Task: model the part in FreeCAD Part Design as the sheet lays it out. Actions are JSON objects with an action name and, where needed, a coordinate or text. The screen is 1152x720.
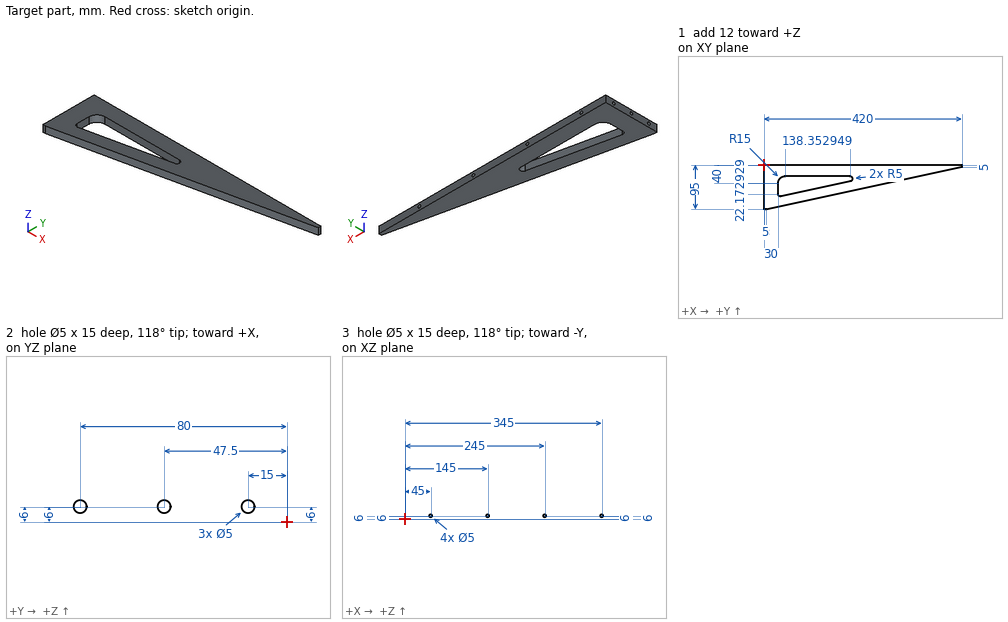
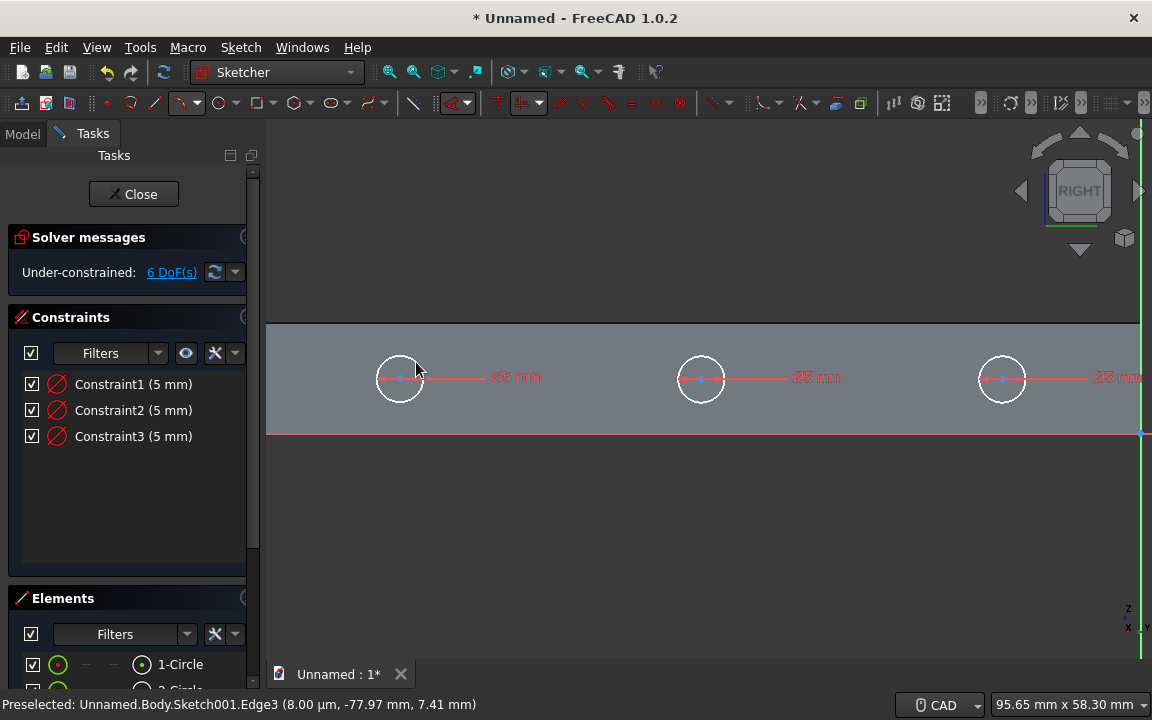
{"action": "scroll", "coordinate": [400, 378], "scroll_direction": "down", "scroll_amount": 2}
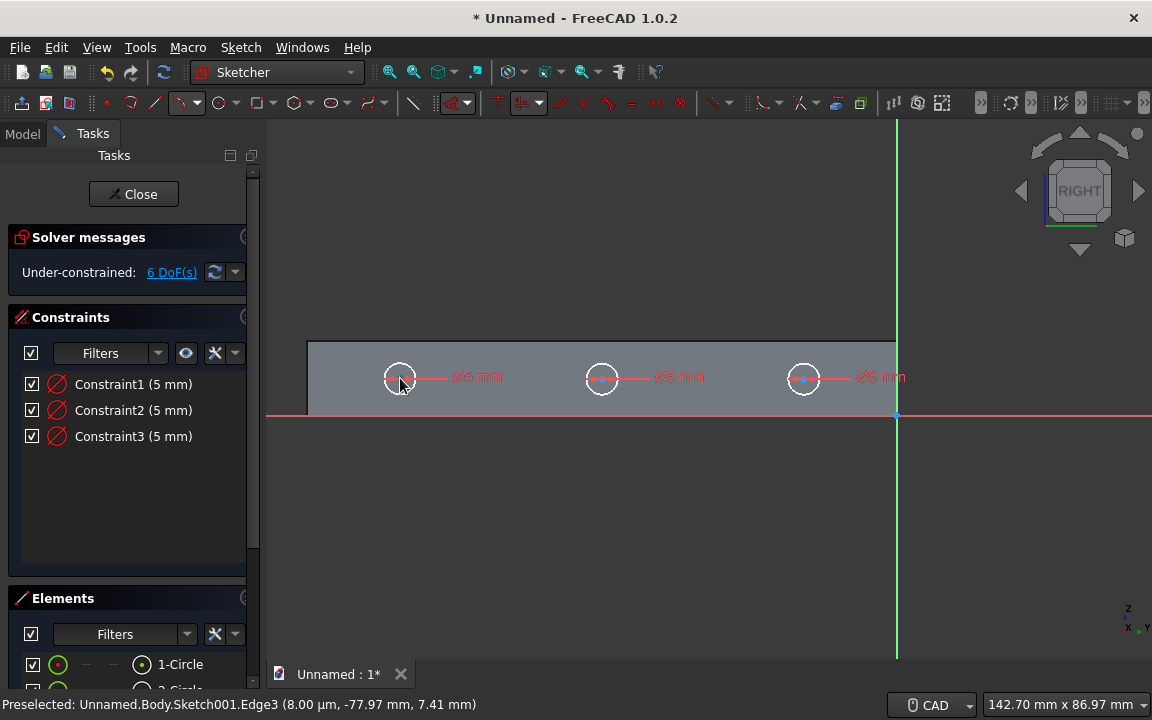
{"action": "left_click", "coordinate": [804, 379]}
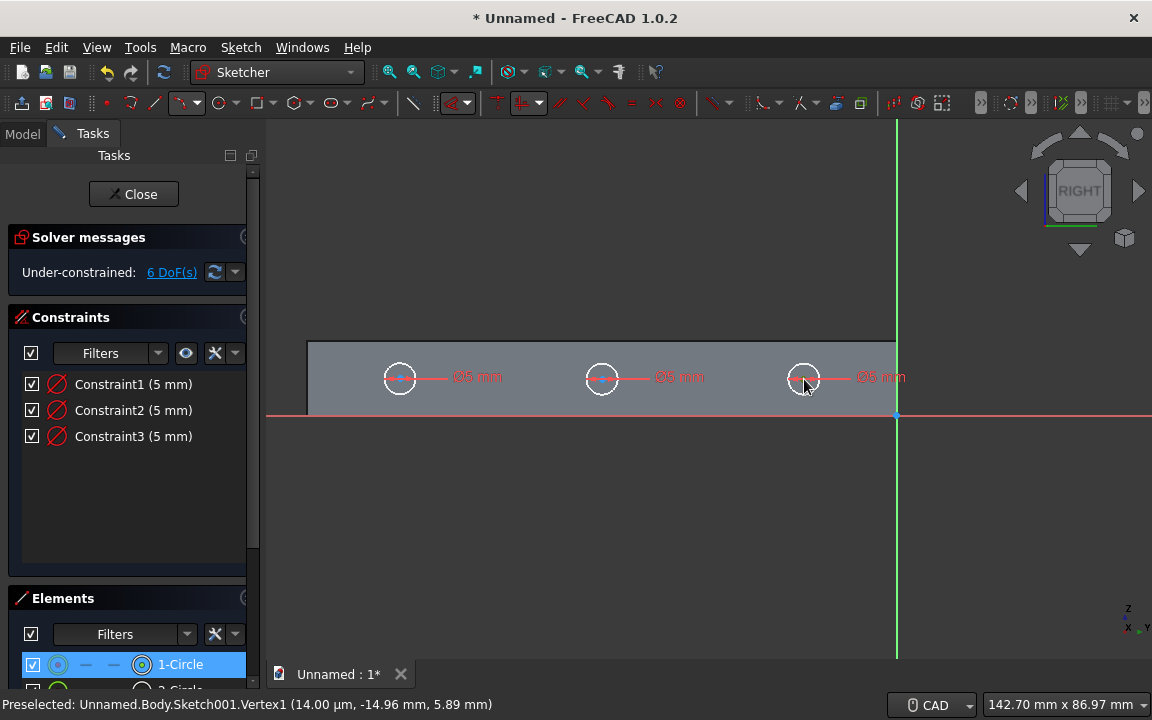
{"action": "left_click", "coordinate": [470, 104]}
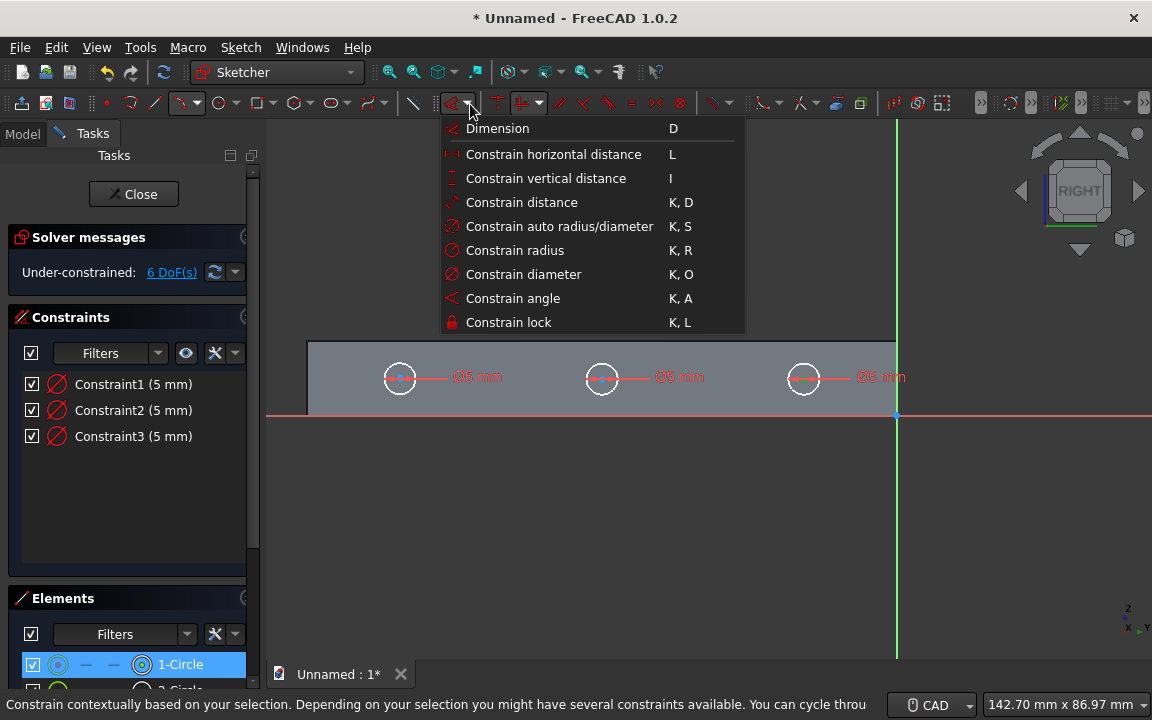
{"action": "left_click", "coordinate": [593, 178]}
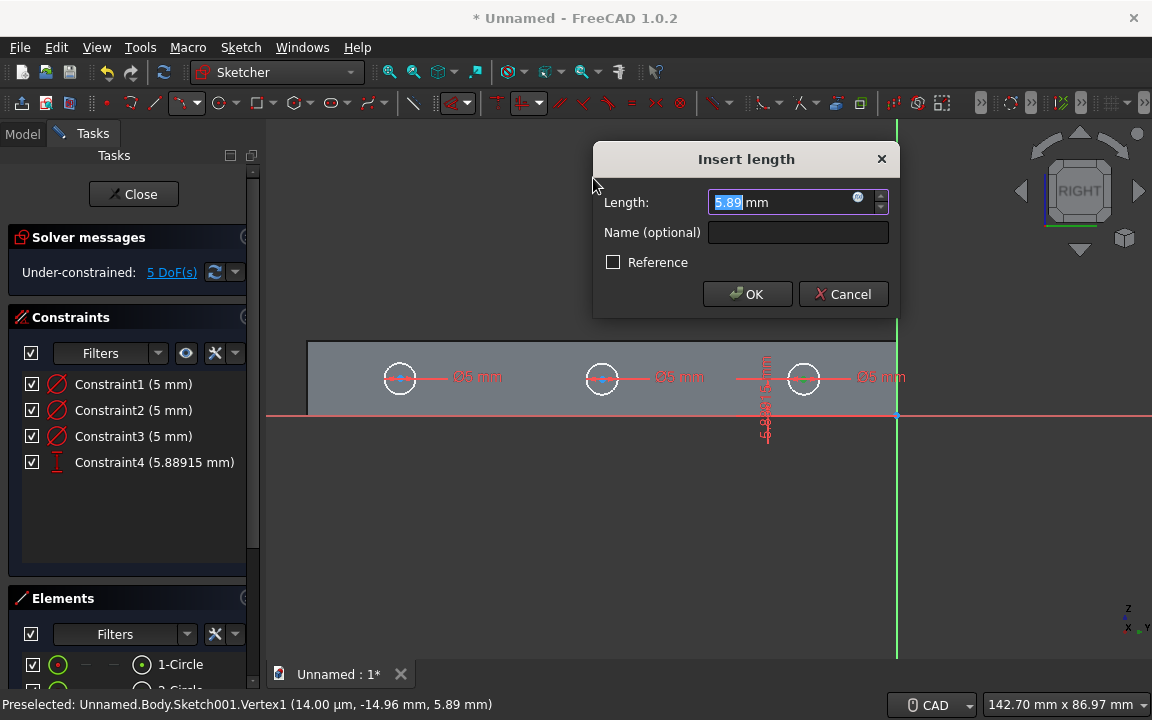
{"action": "type", "text": "6"}
{"action": "key", "text": "Return"}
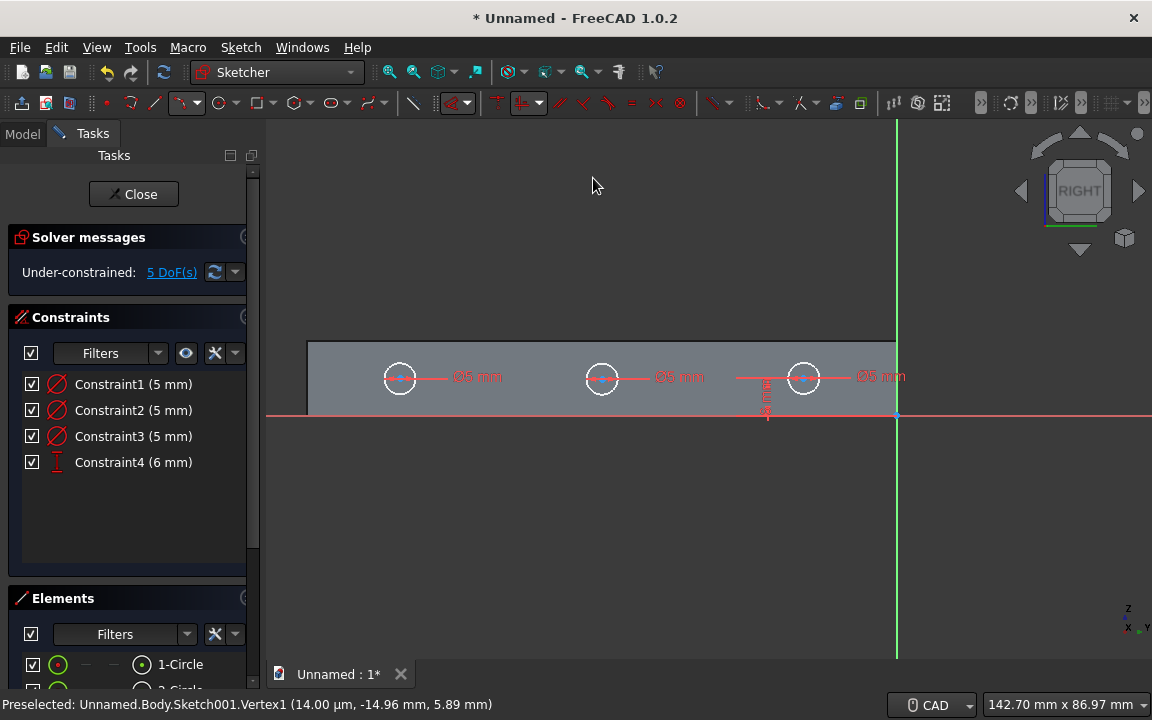
{"action": "left_click", "coordinate": [602, 379]}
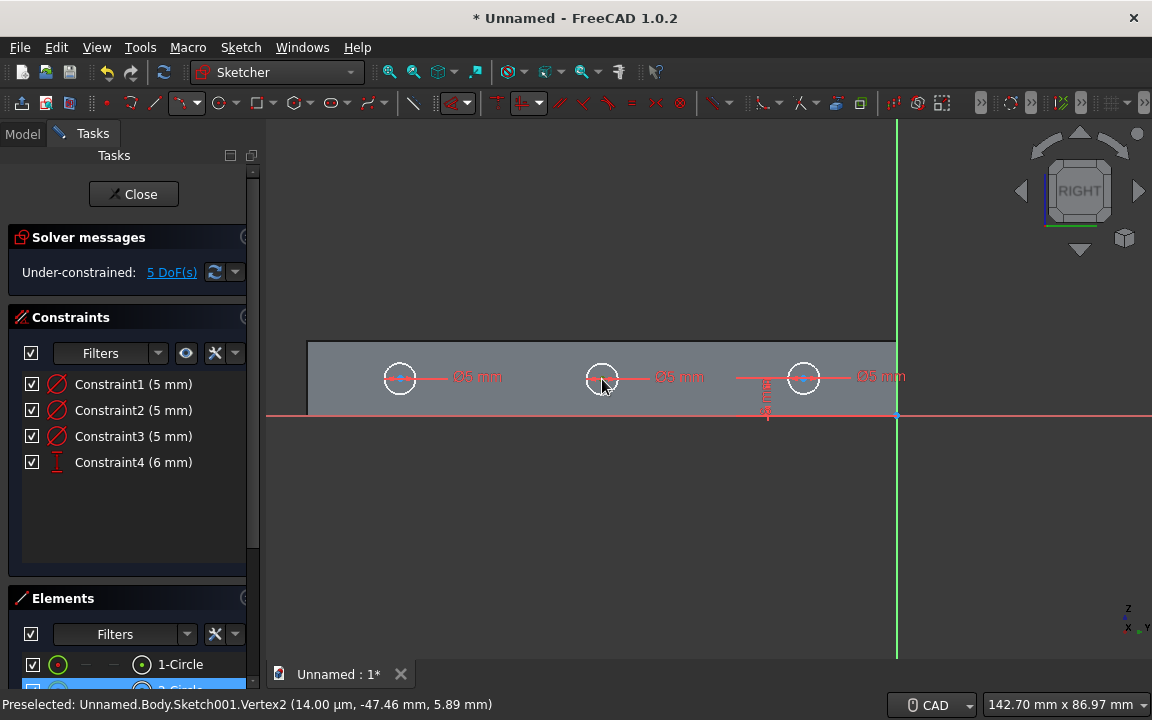
{"action": "left_click", "coordinate": [470, 104]}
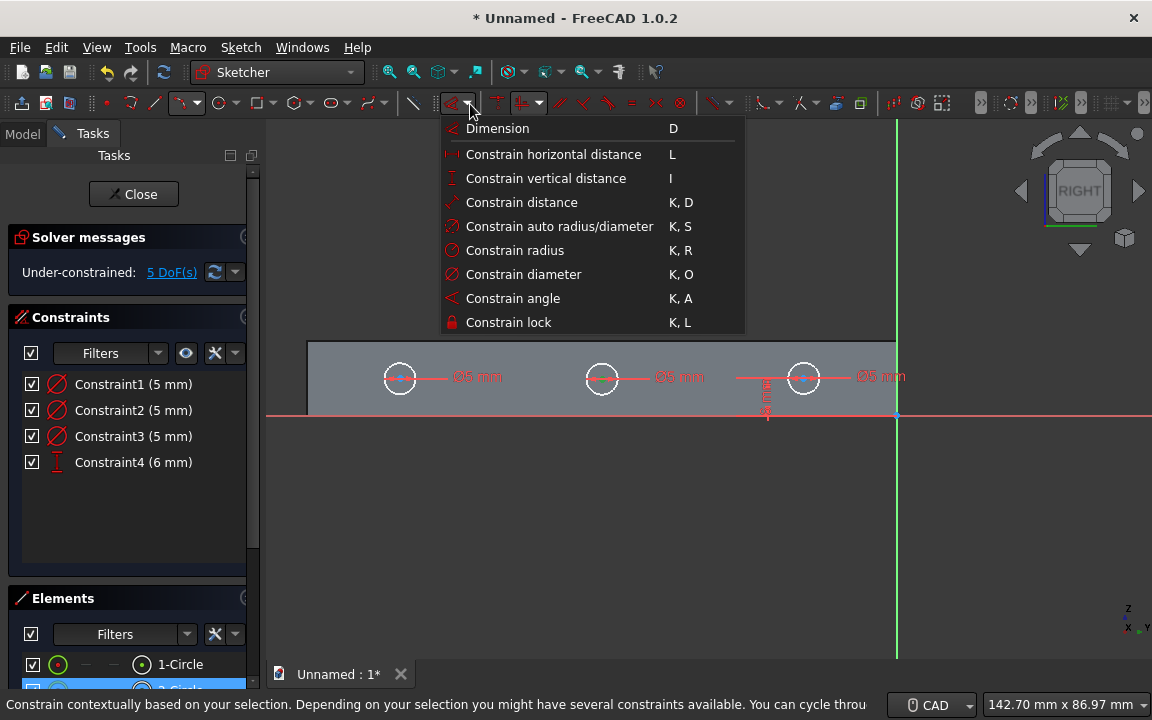
{"action": "left_click", "coordinate": [593, 178]}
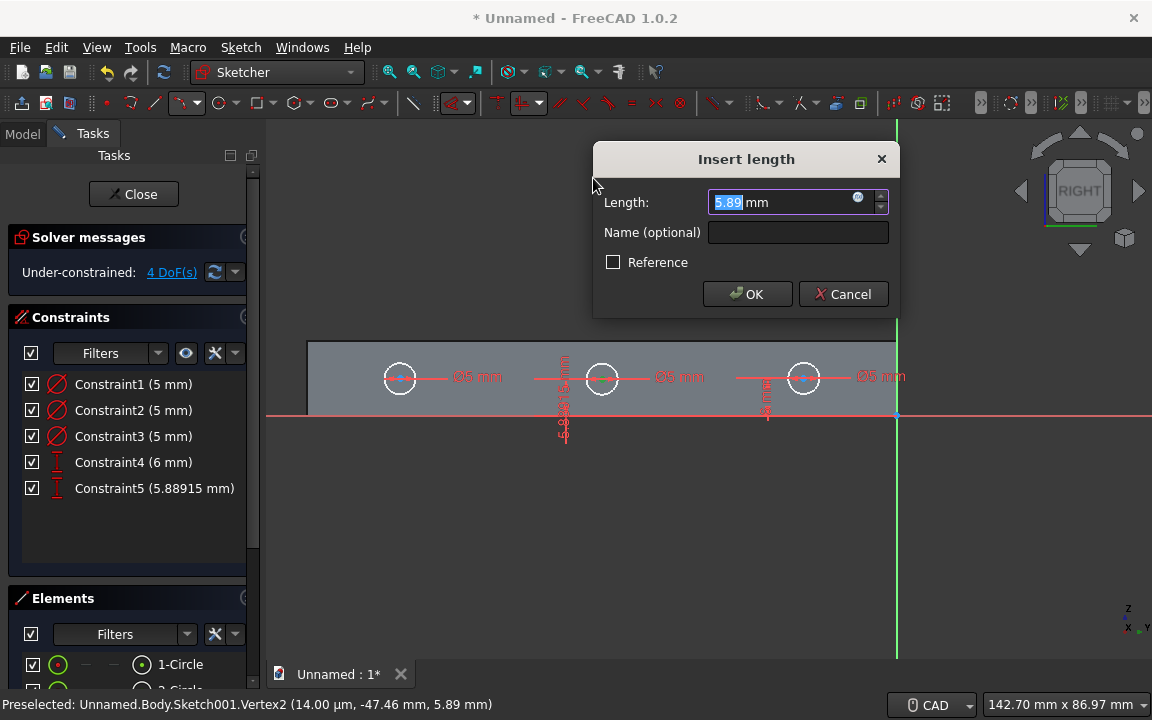
{"action": "type", "text": "6"}
{"action": "key", "text": "Return"}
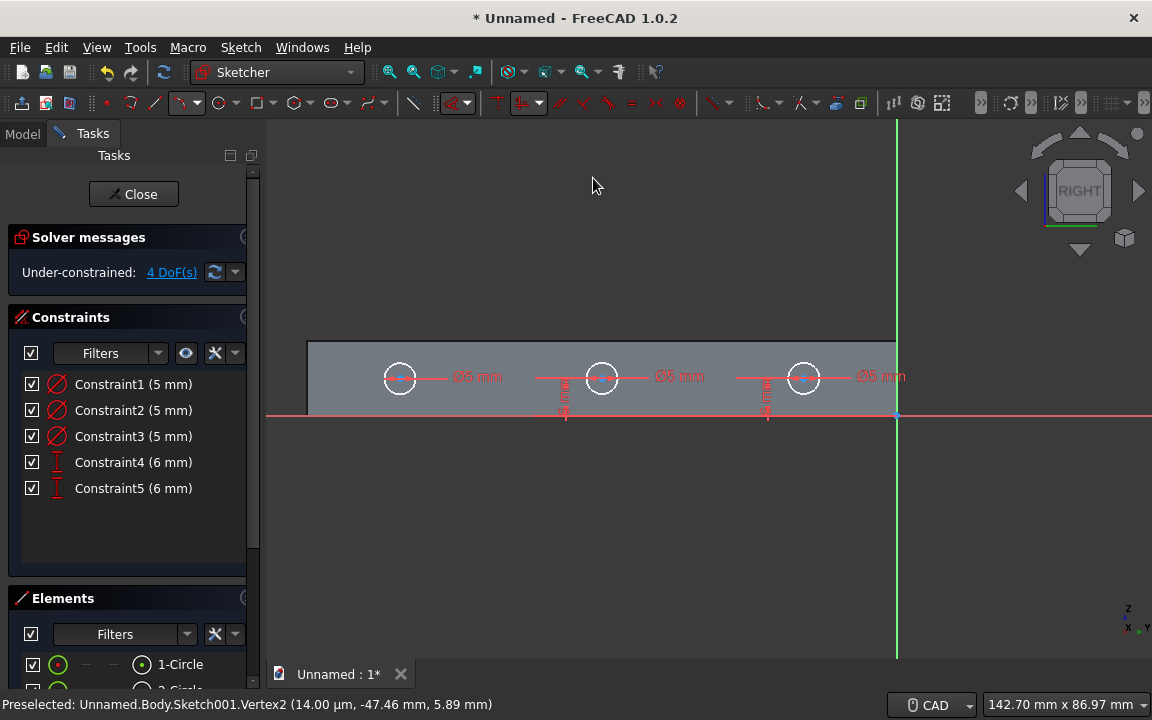
{"action": "left_click", "coordinate": [400, 379]}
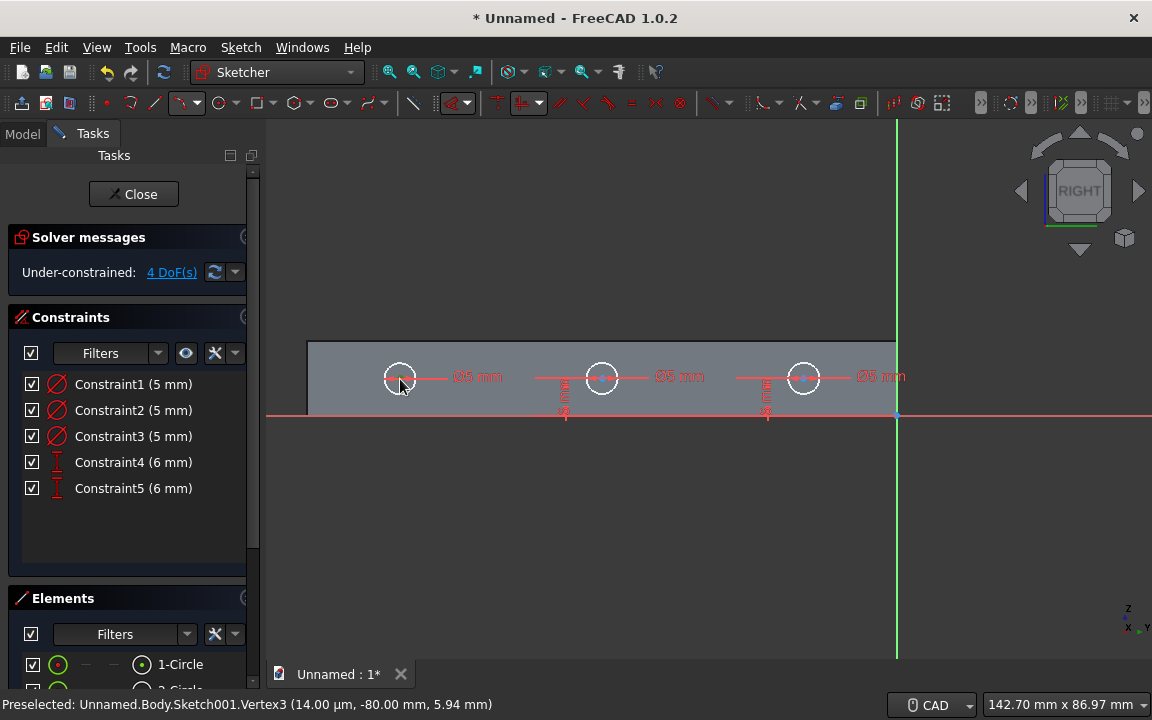
{"action": "left_click", "coordinate": [470, 104]}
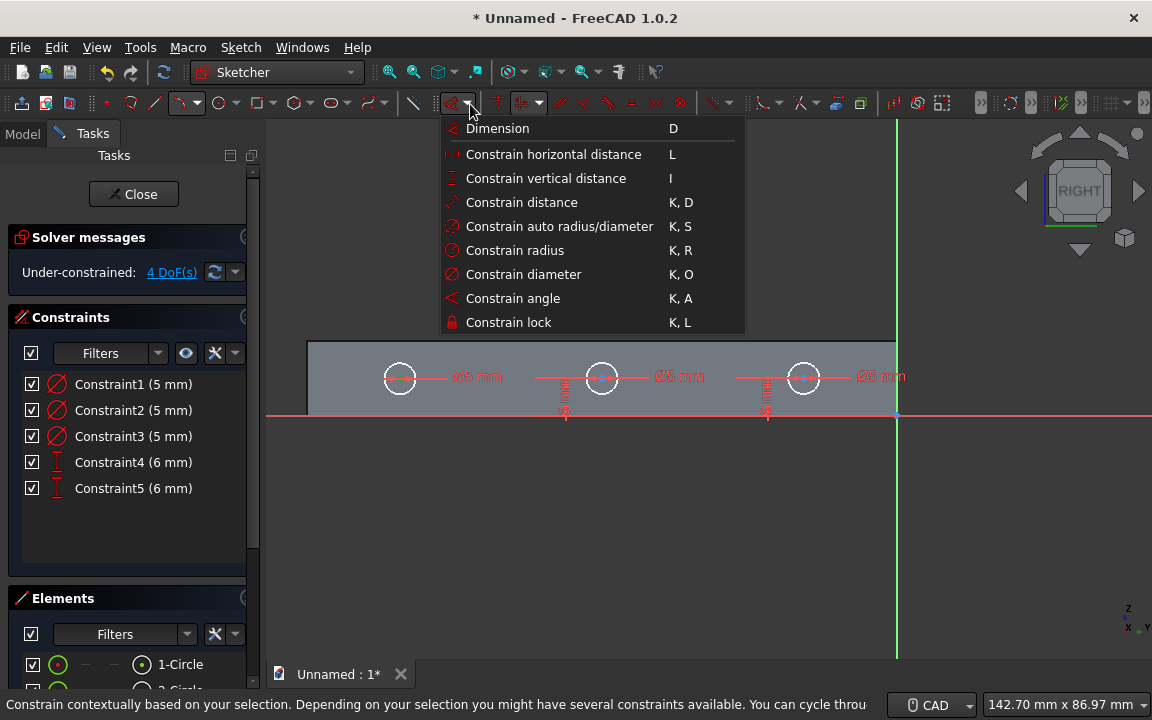
{"action": "left_click", "coordinate": [593, 178]}